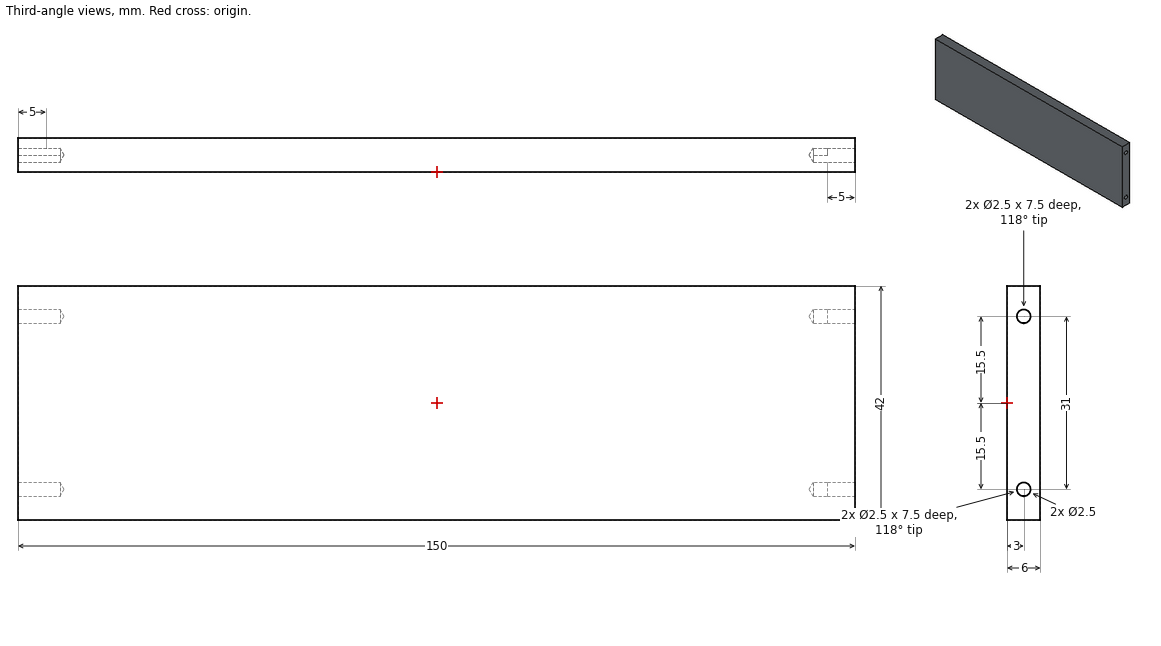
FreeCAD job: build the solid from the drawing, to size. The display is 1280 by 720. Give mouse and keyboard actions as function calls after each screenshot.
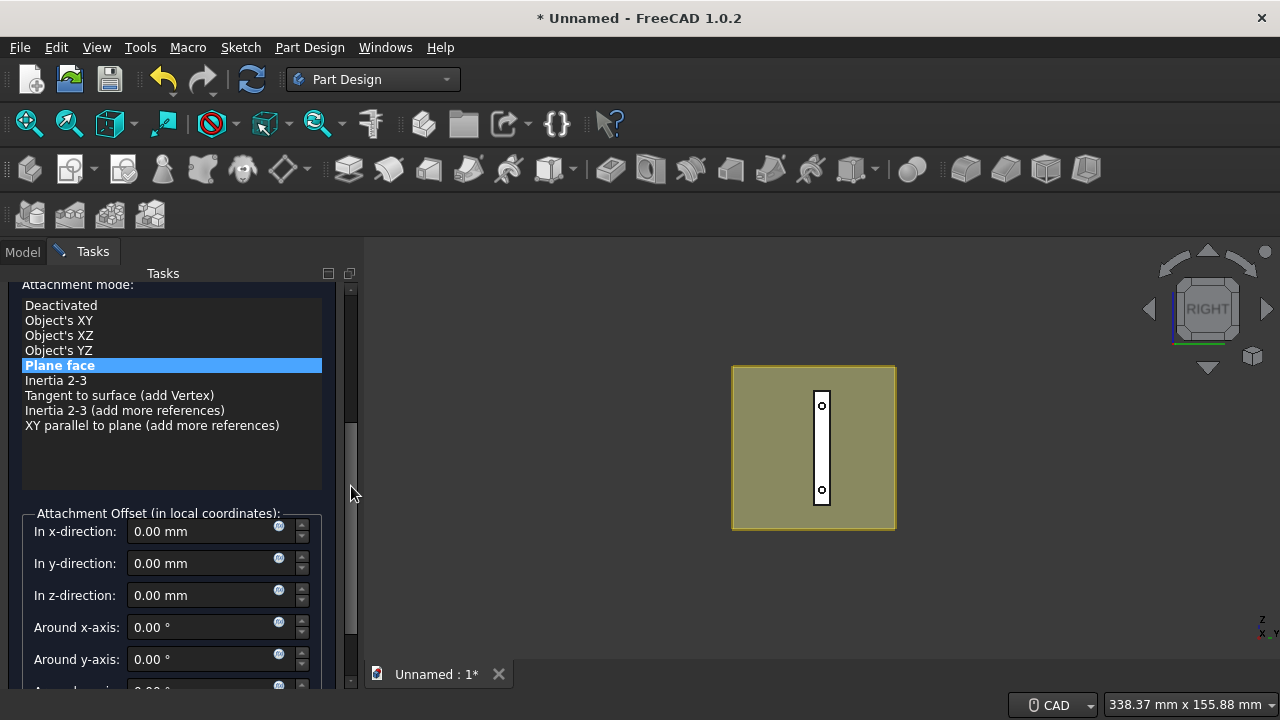
triple_click(210, 595)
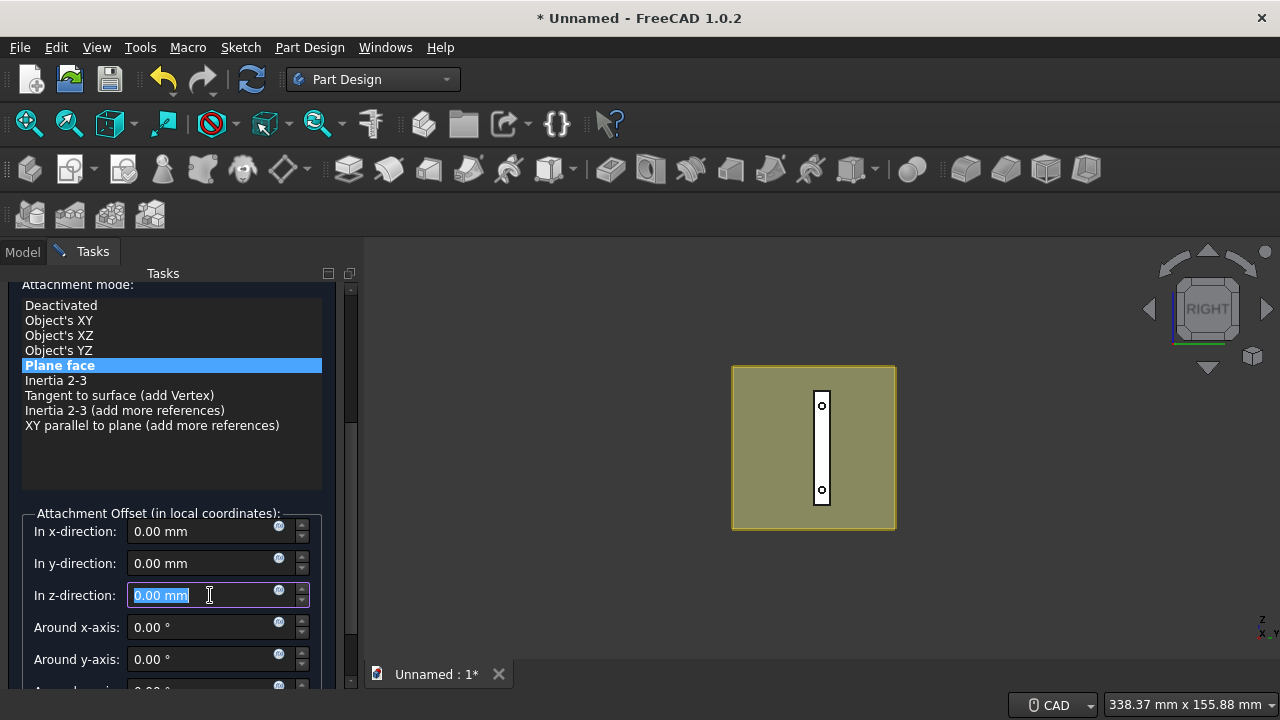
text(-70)
key(Tab)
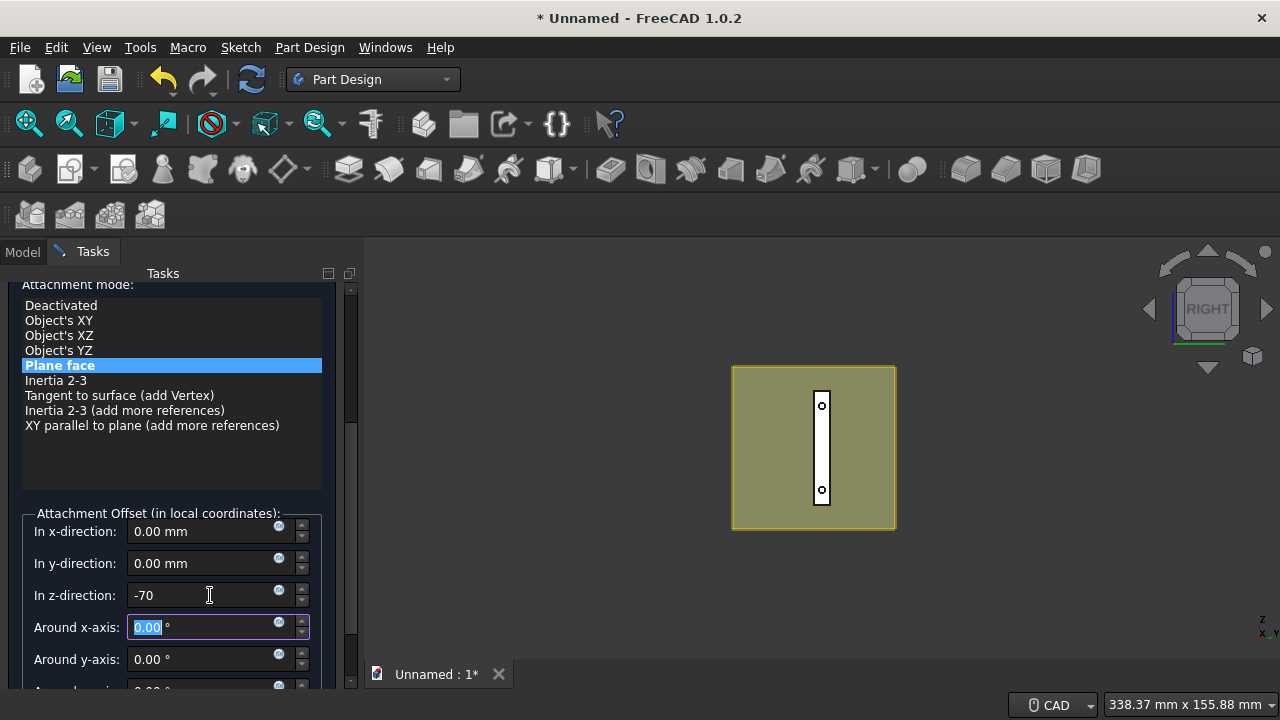
scroll(351, 486, up, 5)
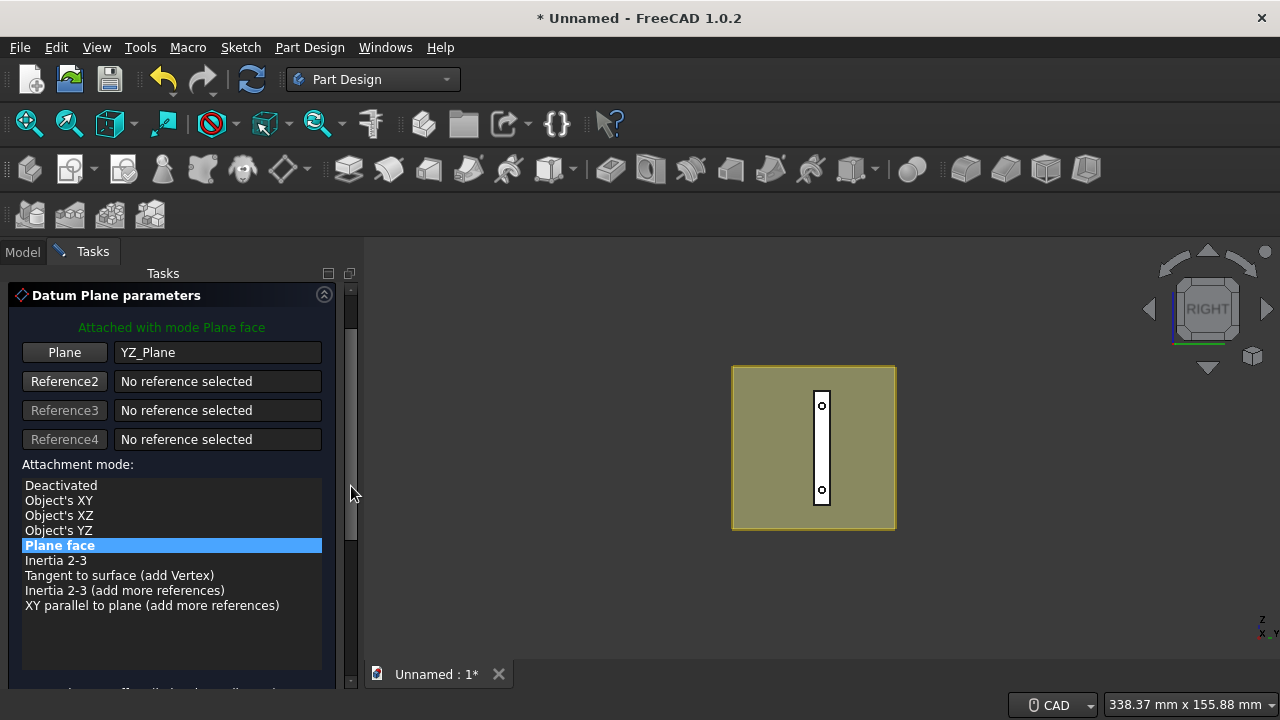
click(124, 312)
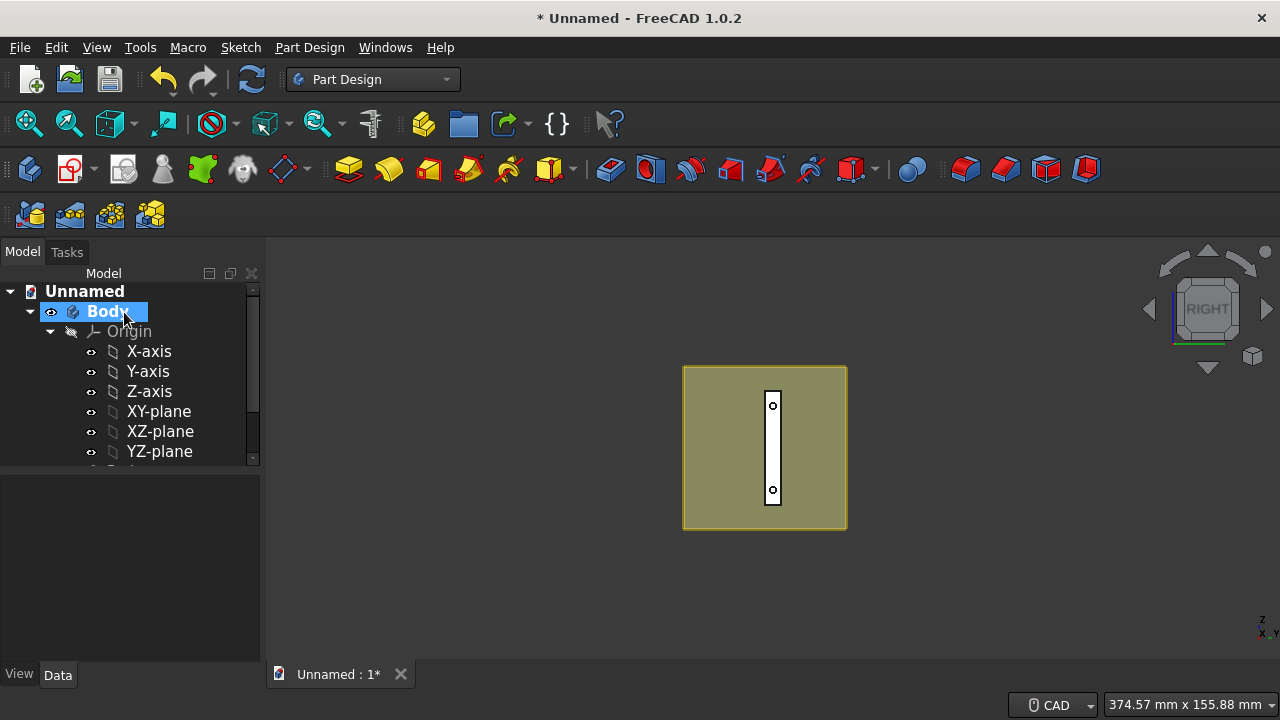
scroll(100, 367, down, 3)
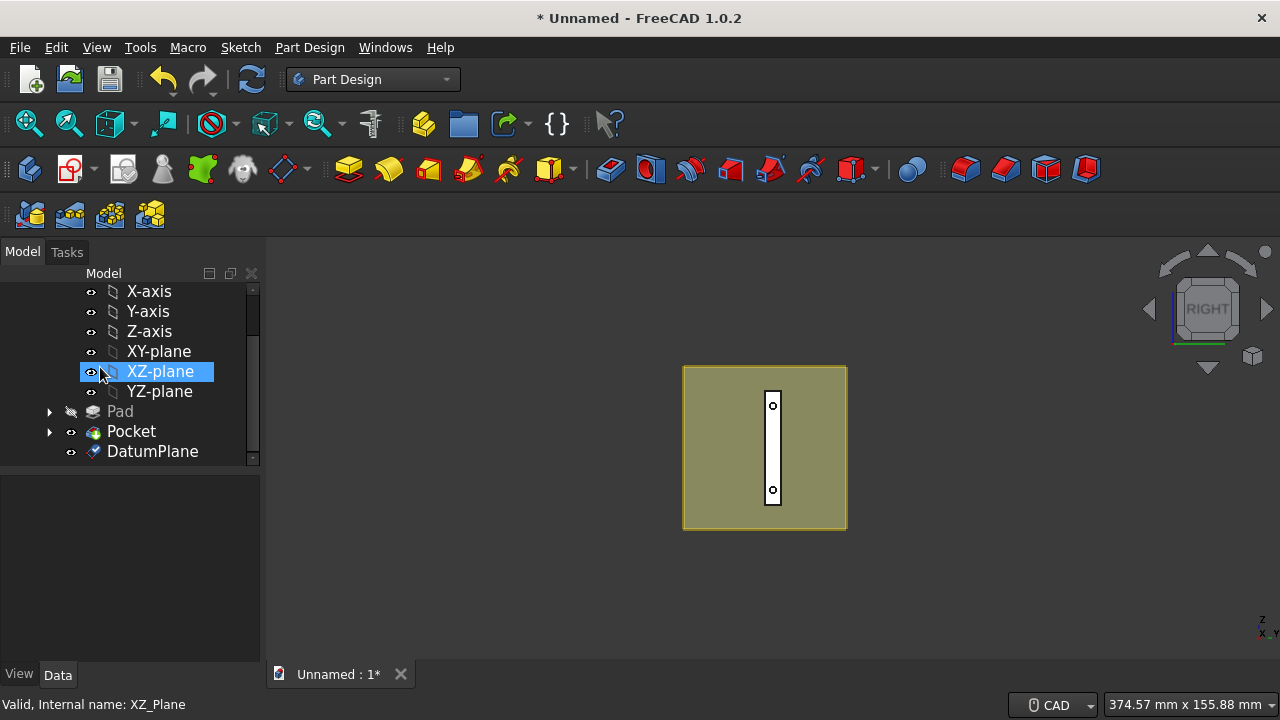
click(116, 452)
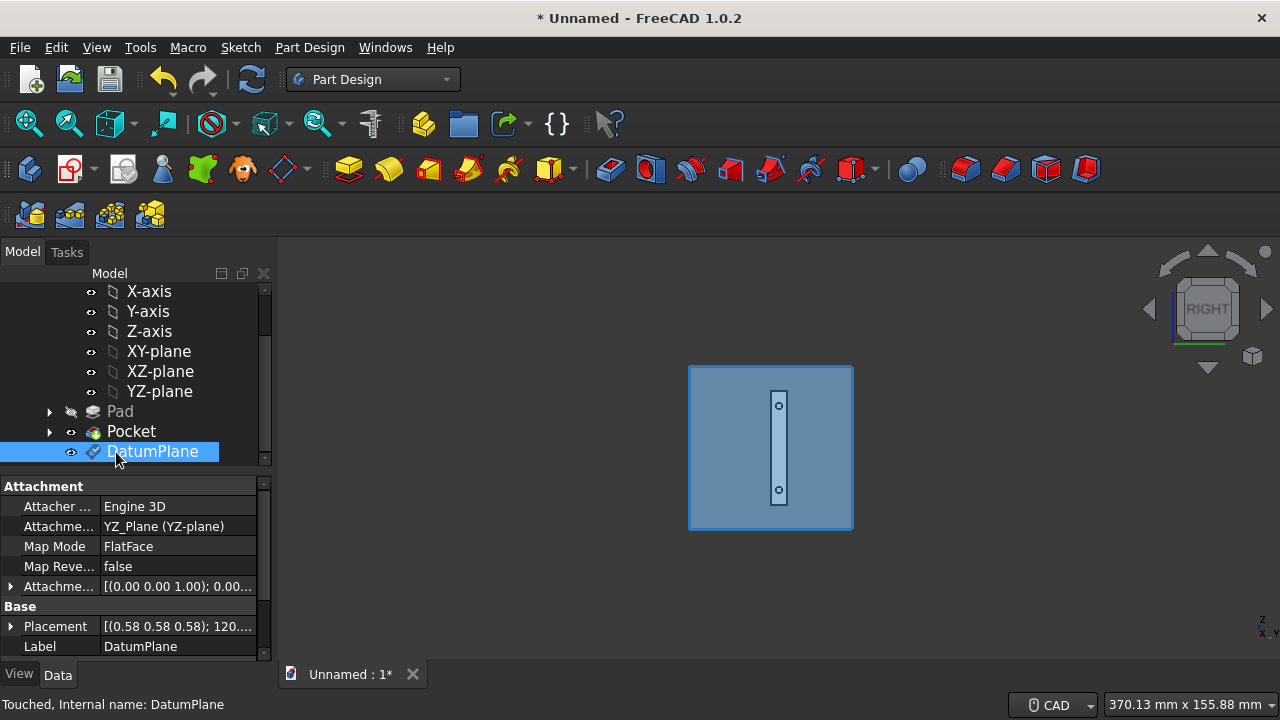
click(70, 170)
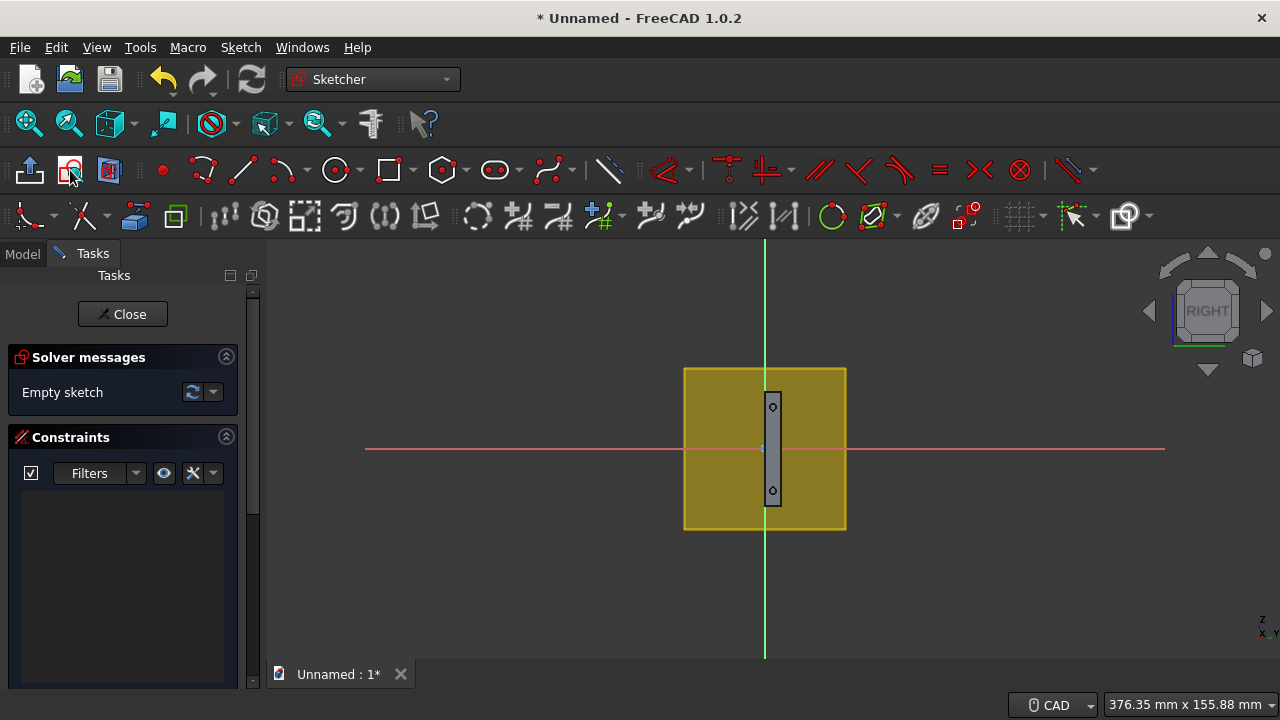
click(110, 170)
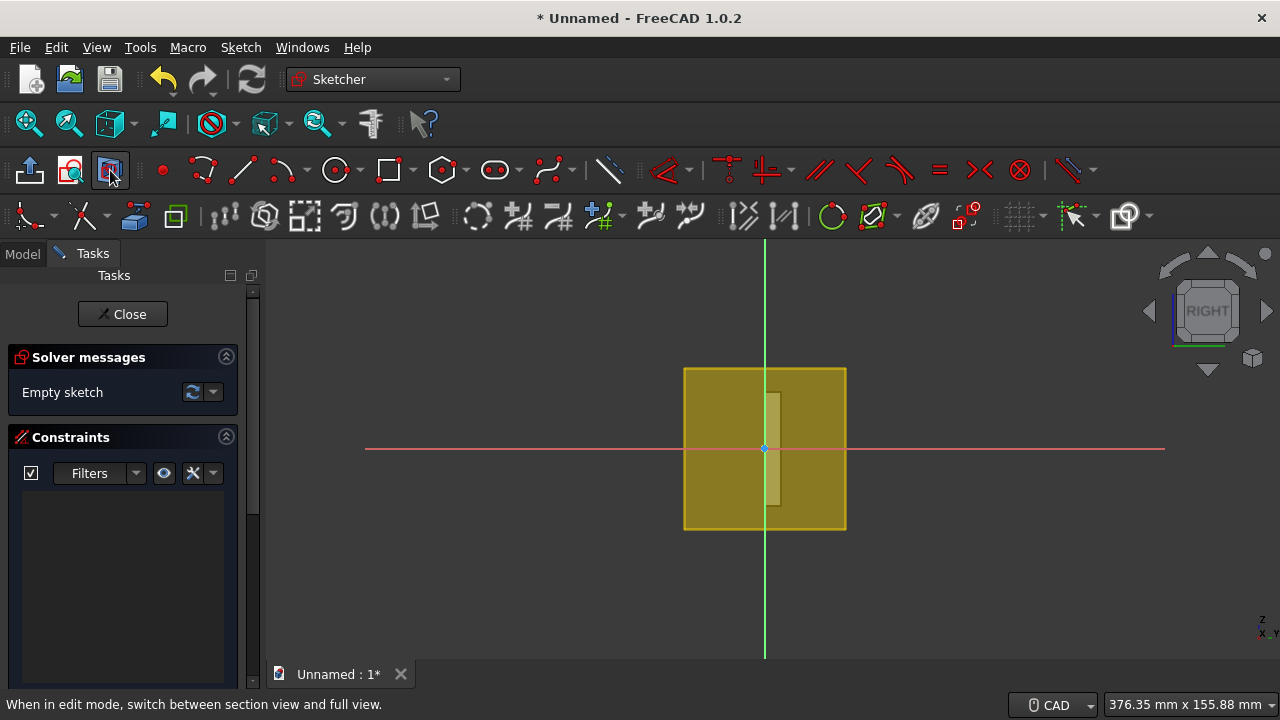
scroll(809, 449, up, 5)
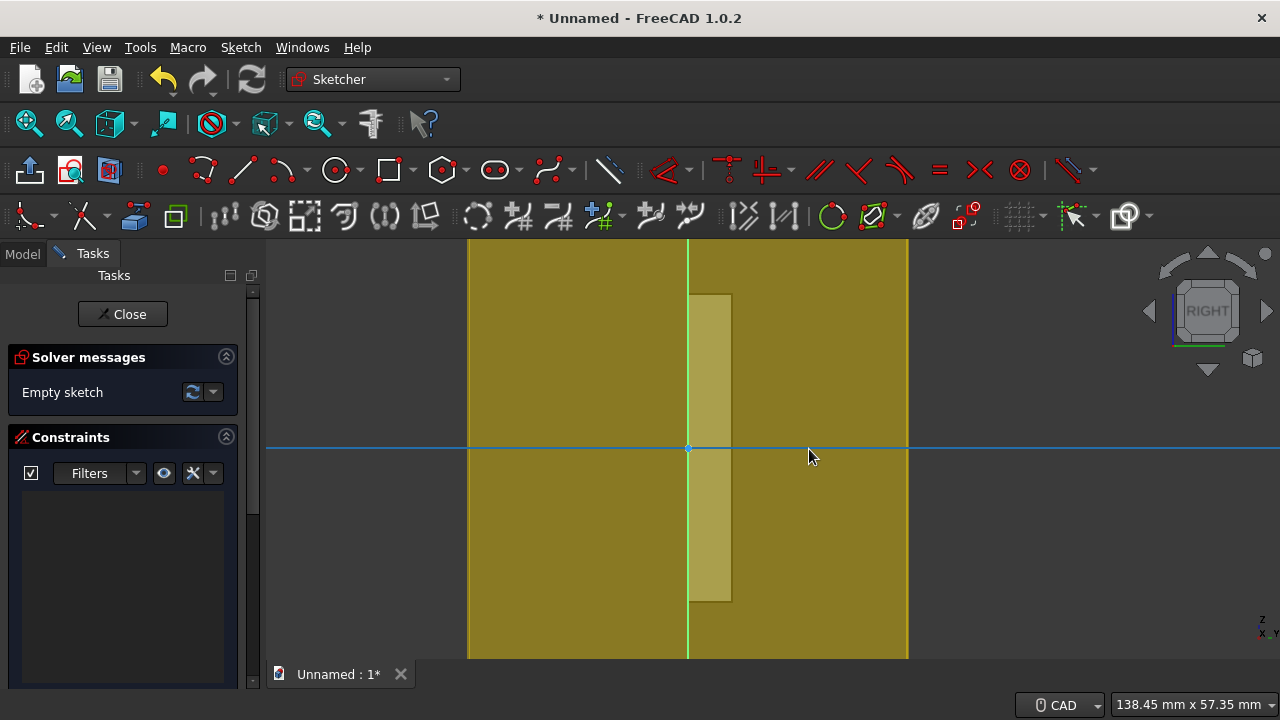
click(336, 170)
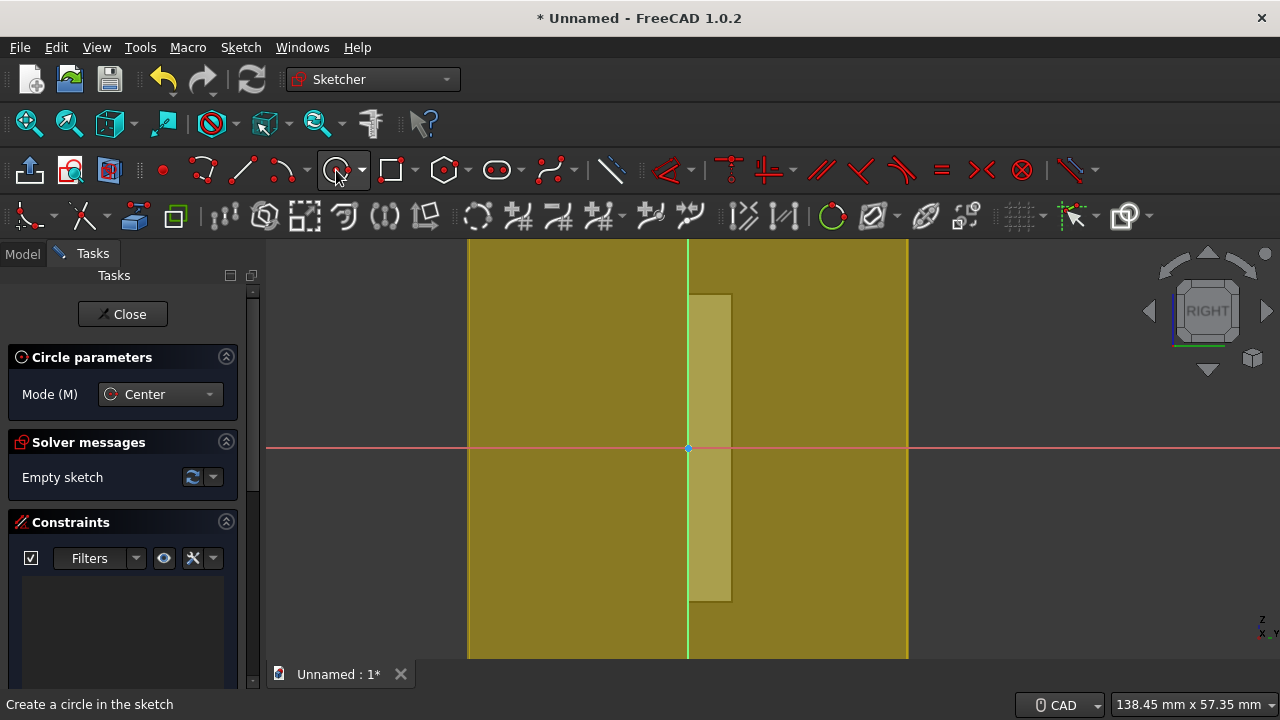
scroll(710, 562, up, 5)